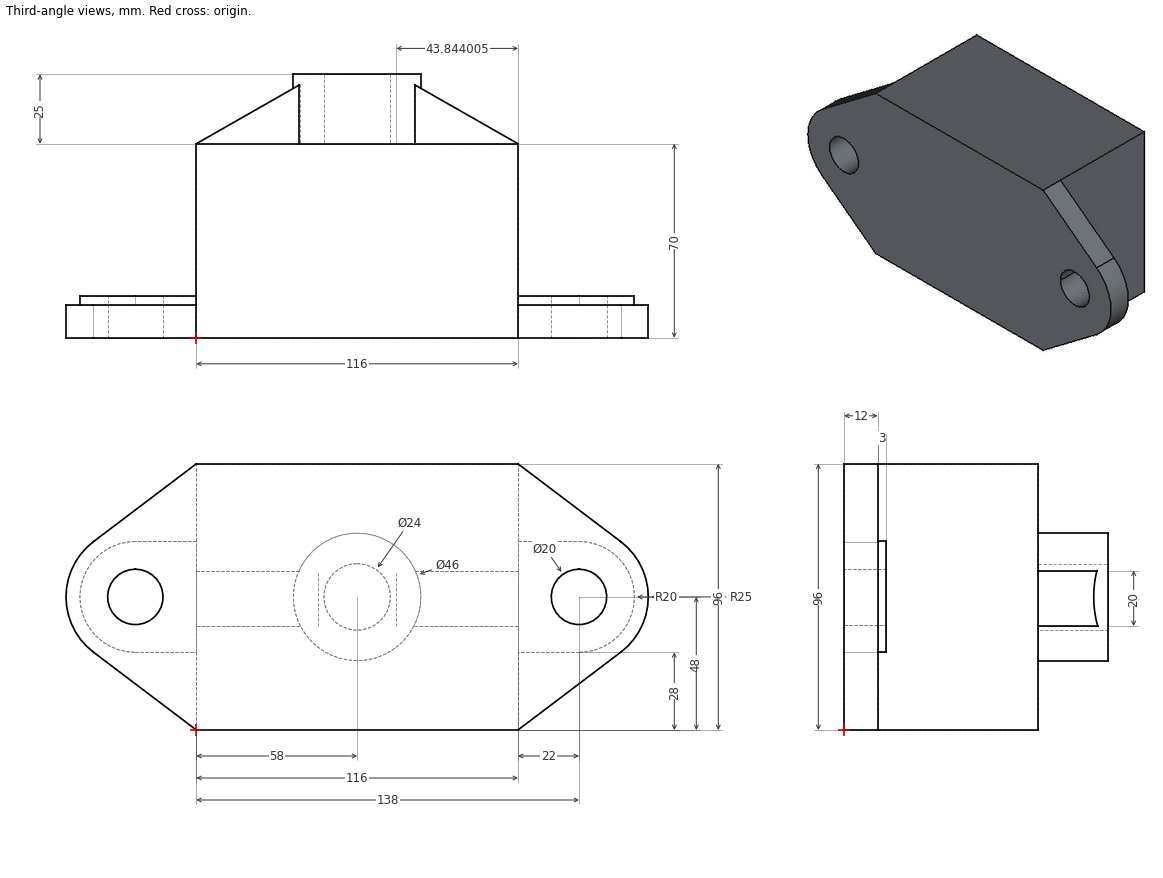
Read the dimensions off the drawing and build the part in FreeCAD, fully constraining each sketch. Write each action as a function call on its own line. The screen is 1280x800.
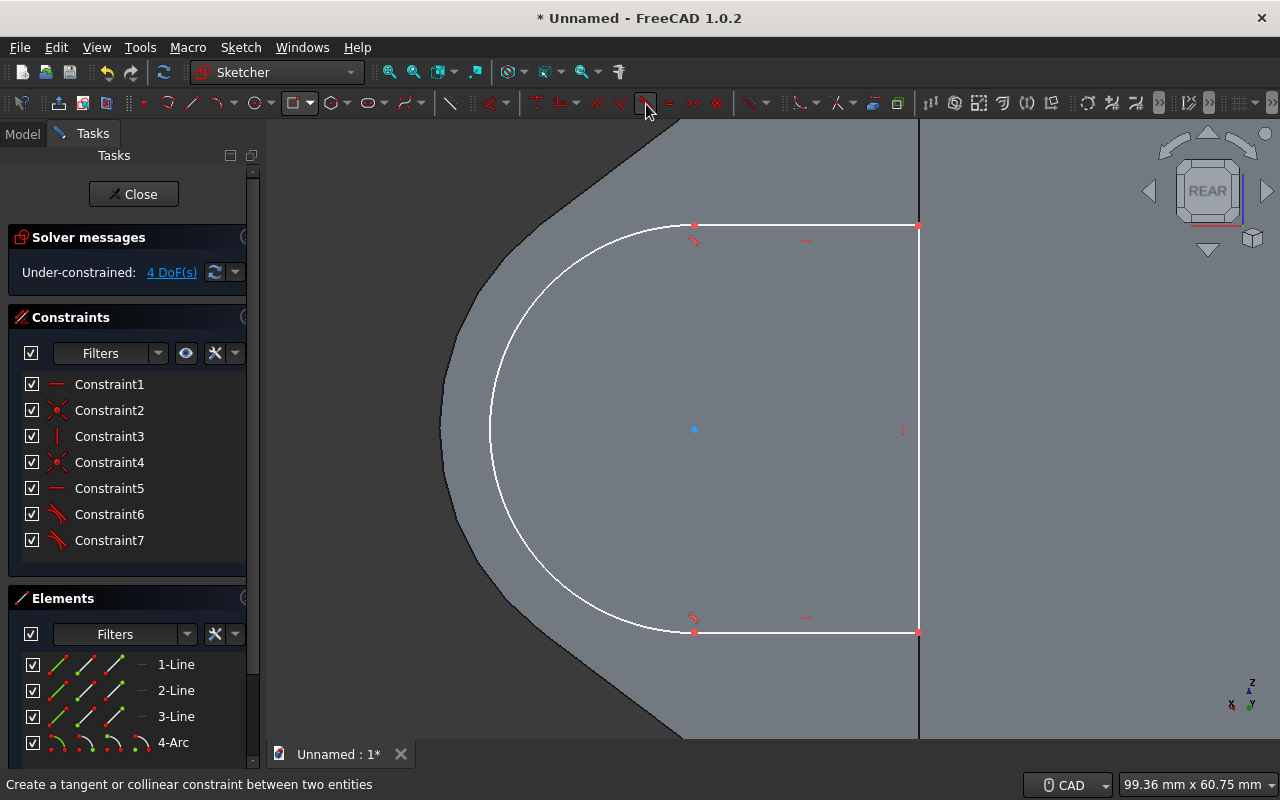
click(490, 104)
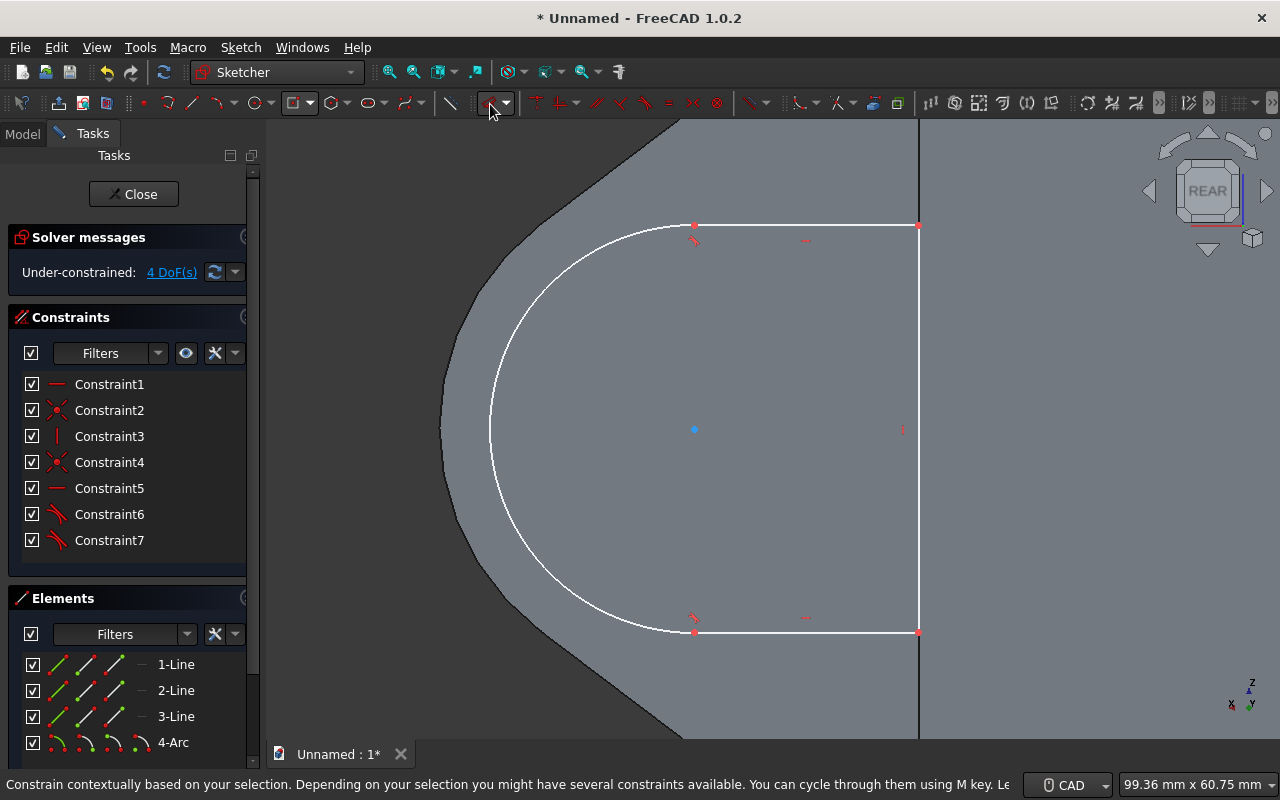
click(529, 309)
click(503, 290)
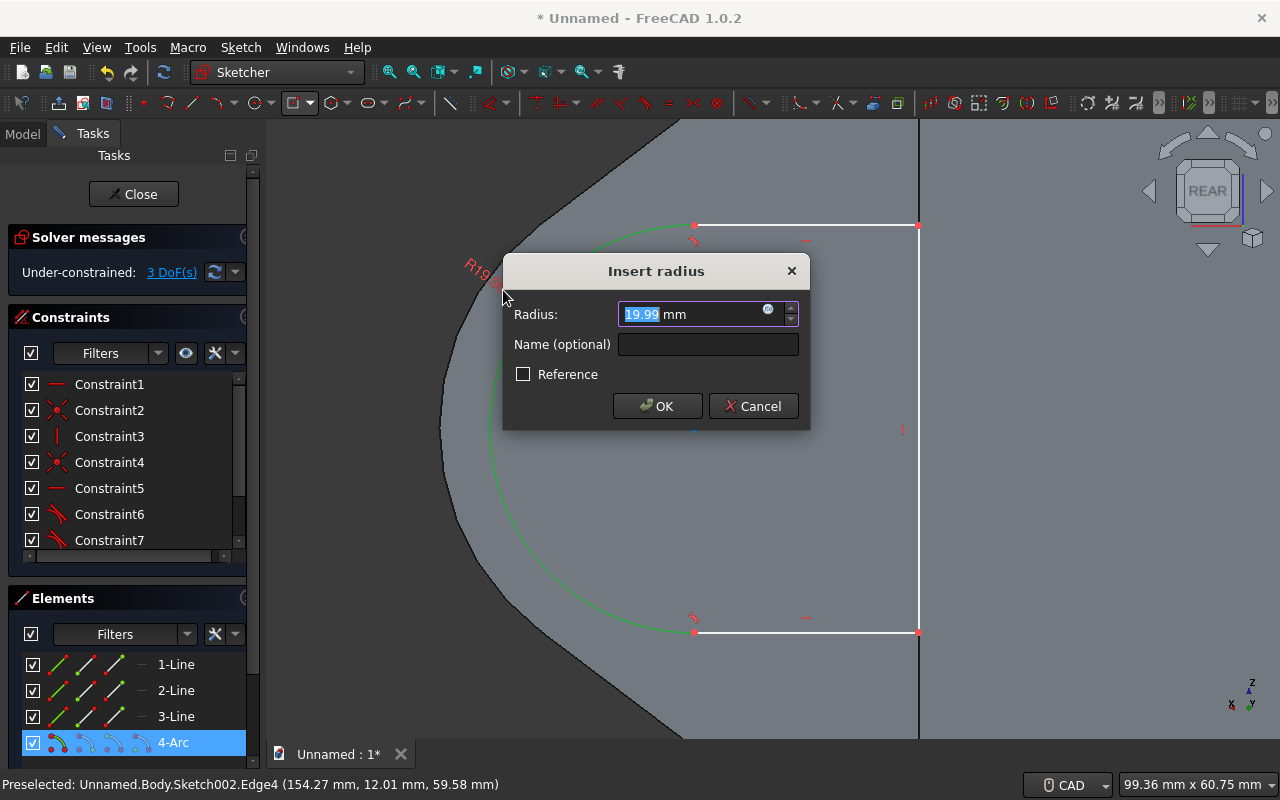
text(20)
key(Return)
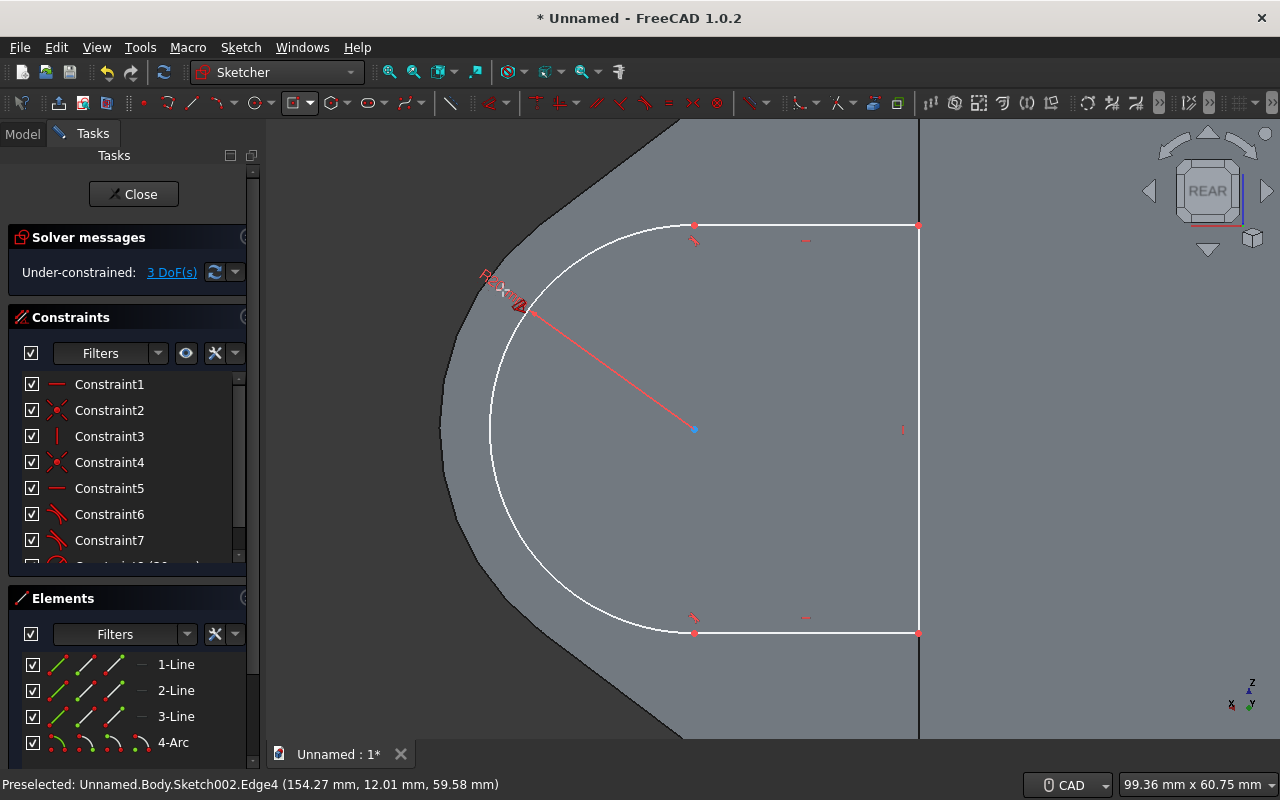
click(762, 633)
click(807, 667)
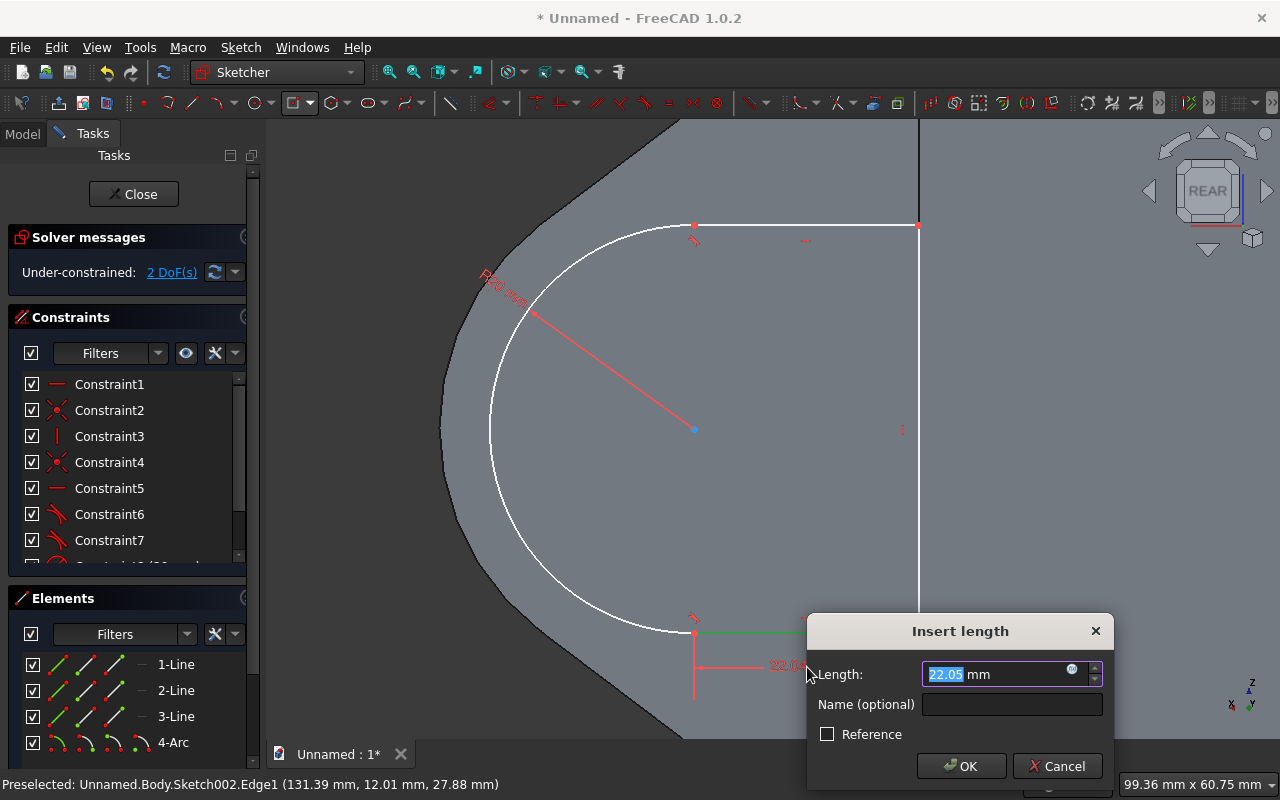
text(22)
key(Return)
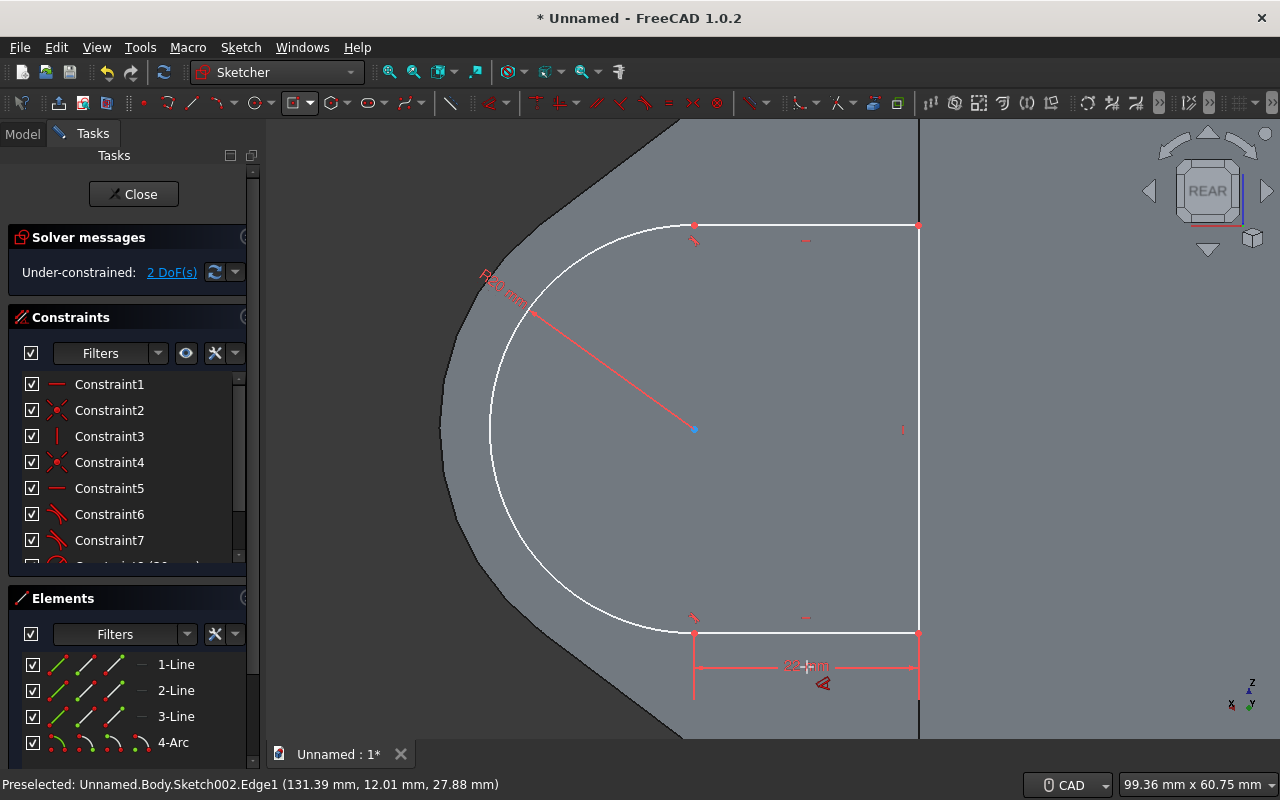
click(694, 633)
click(660, 672)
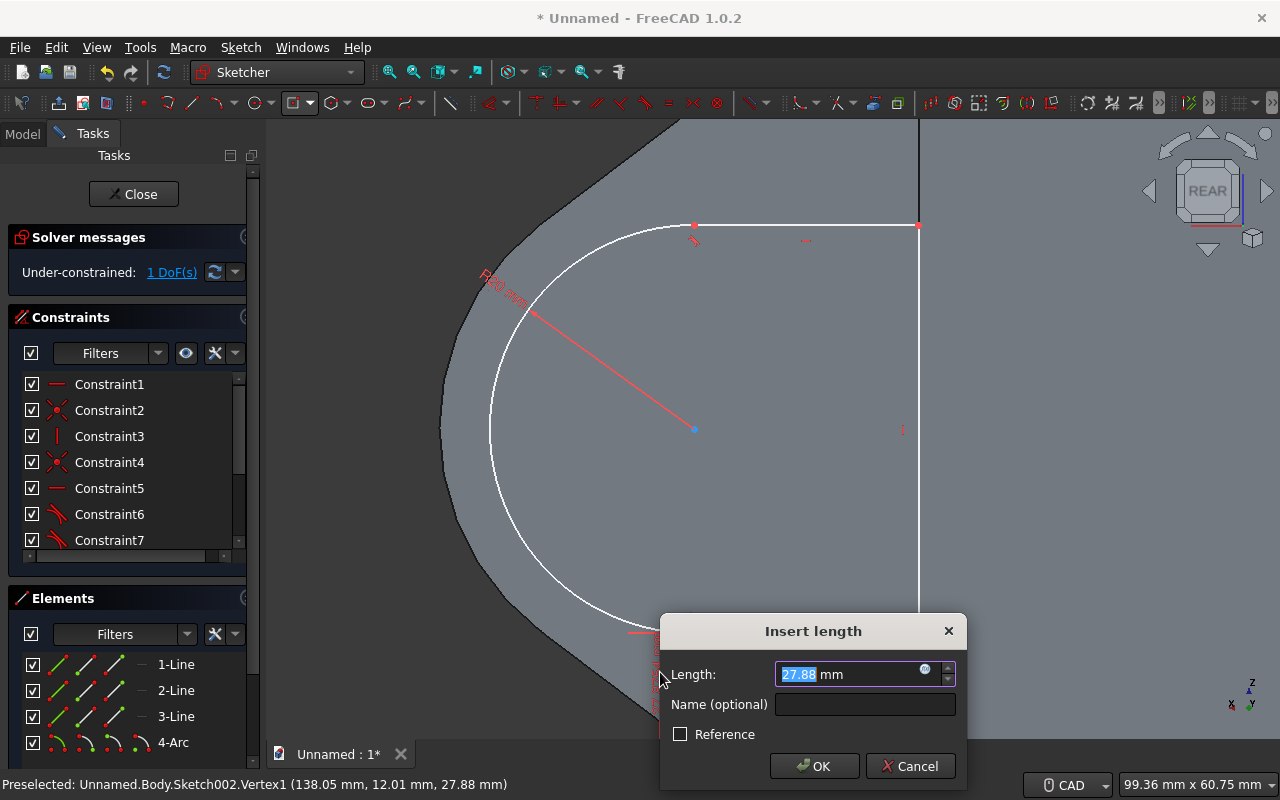
text(28)
key(Return)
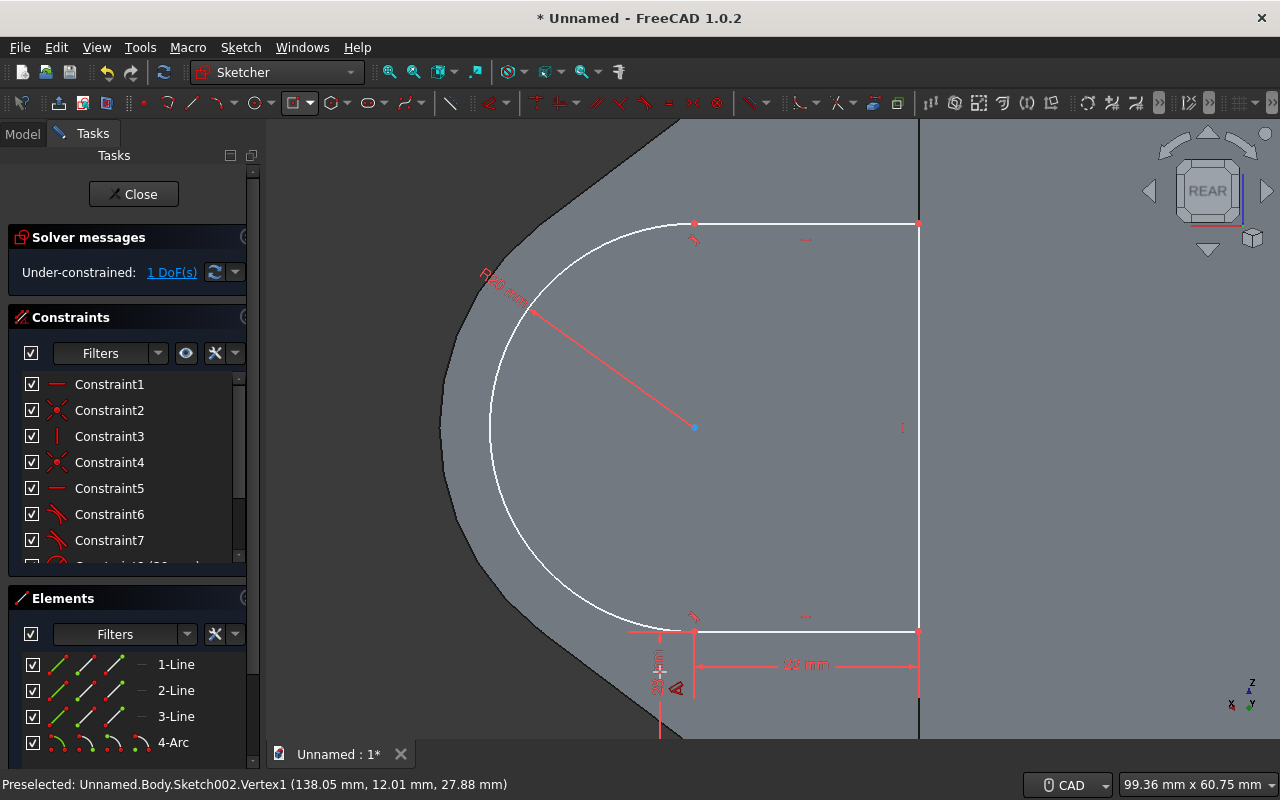
click(694, 632)
click(905, 598)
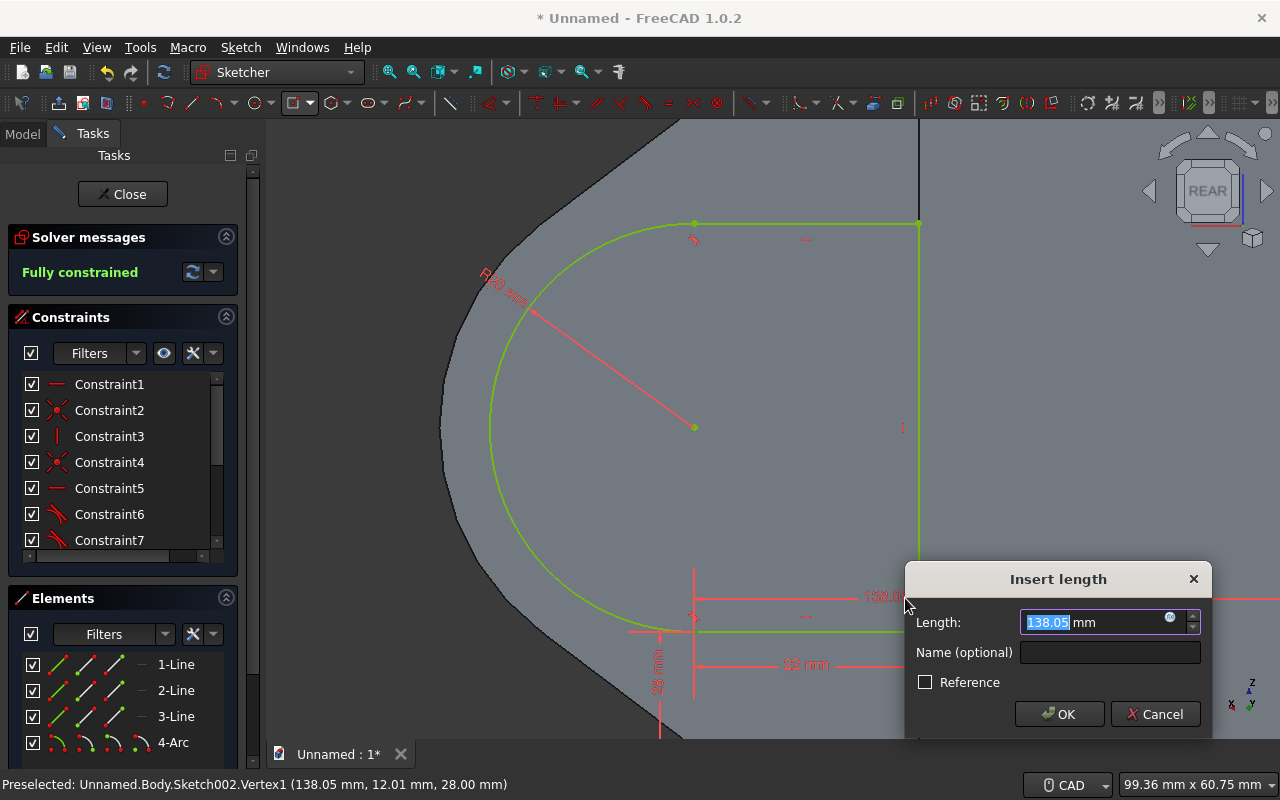
text(138)
key(Return)
key(Escape)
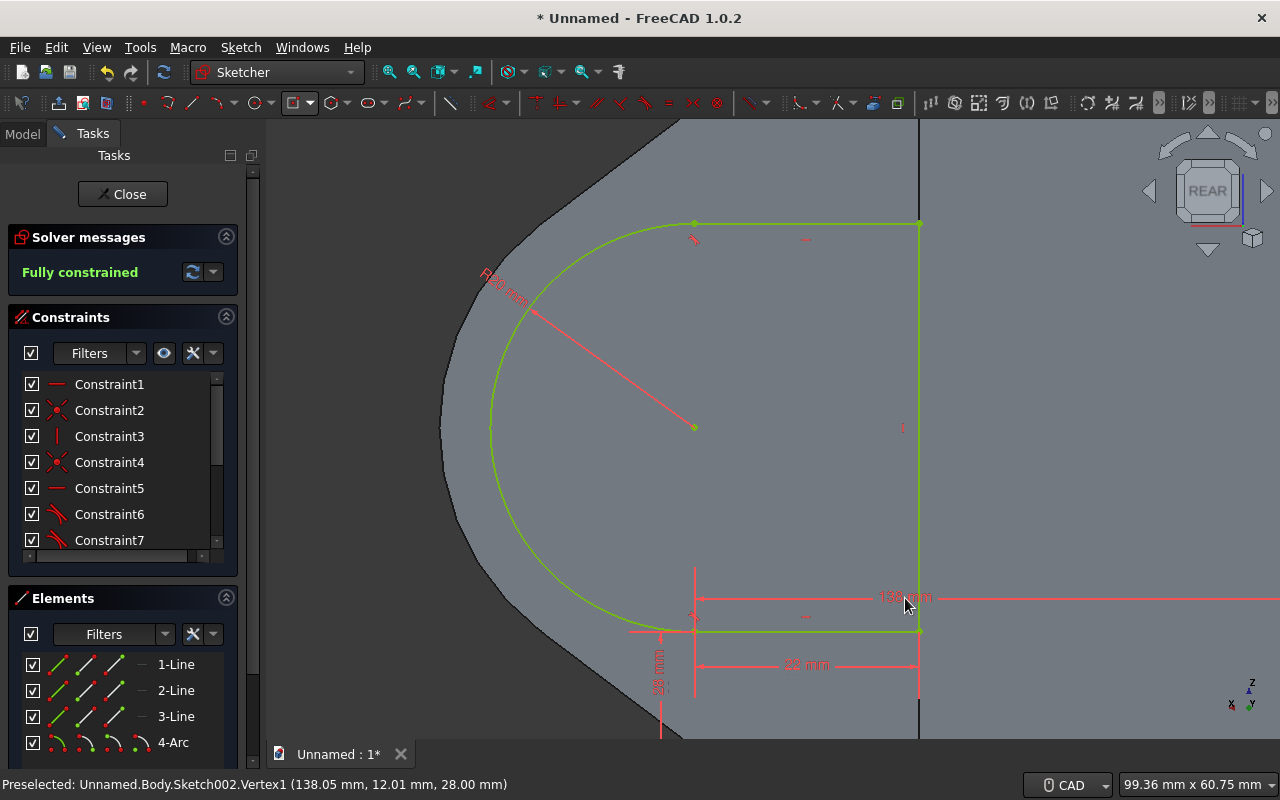
click(123, 194)